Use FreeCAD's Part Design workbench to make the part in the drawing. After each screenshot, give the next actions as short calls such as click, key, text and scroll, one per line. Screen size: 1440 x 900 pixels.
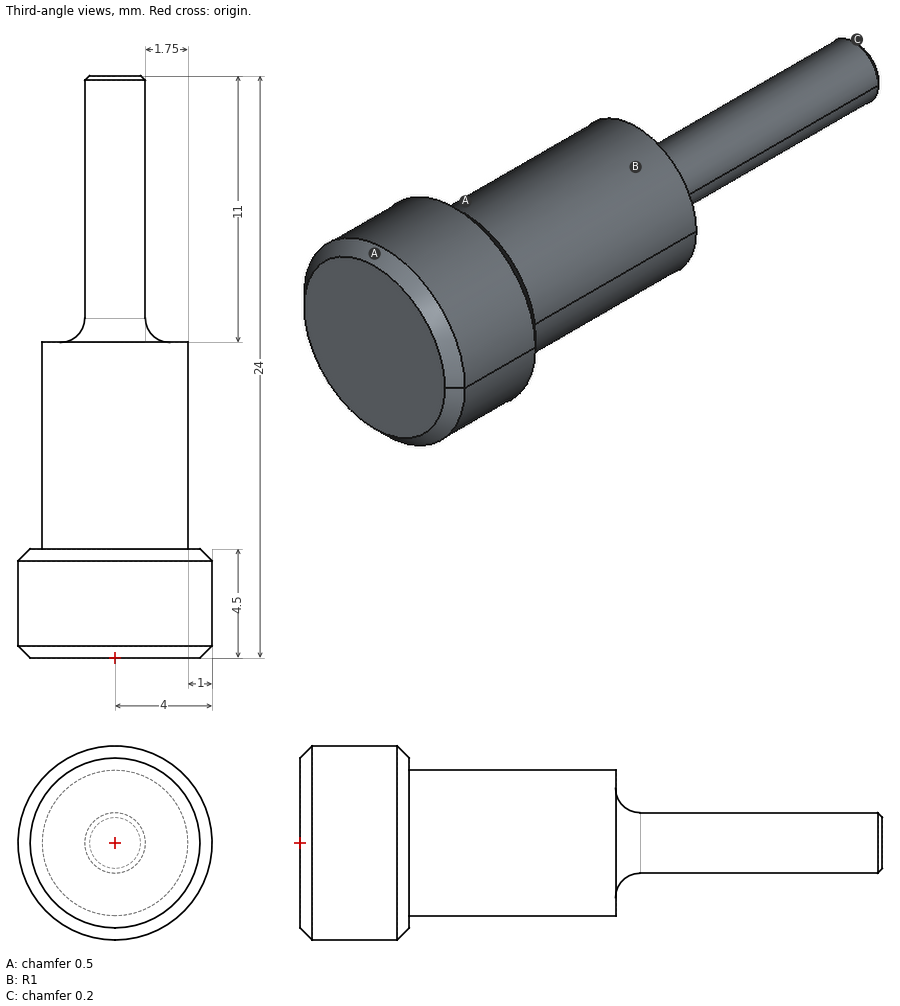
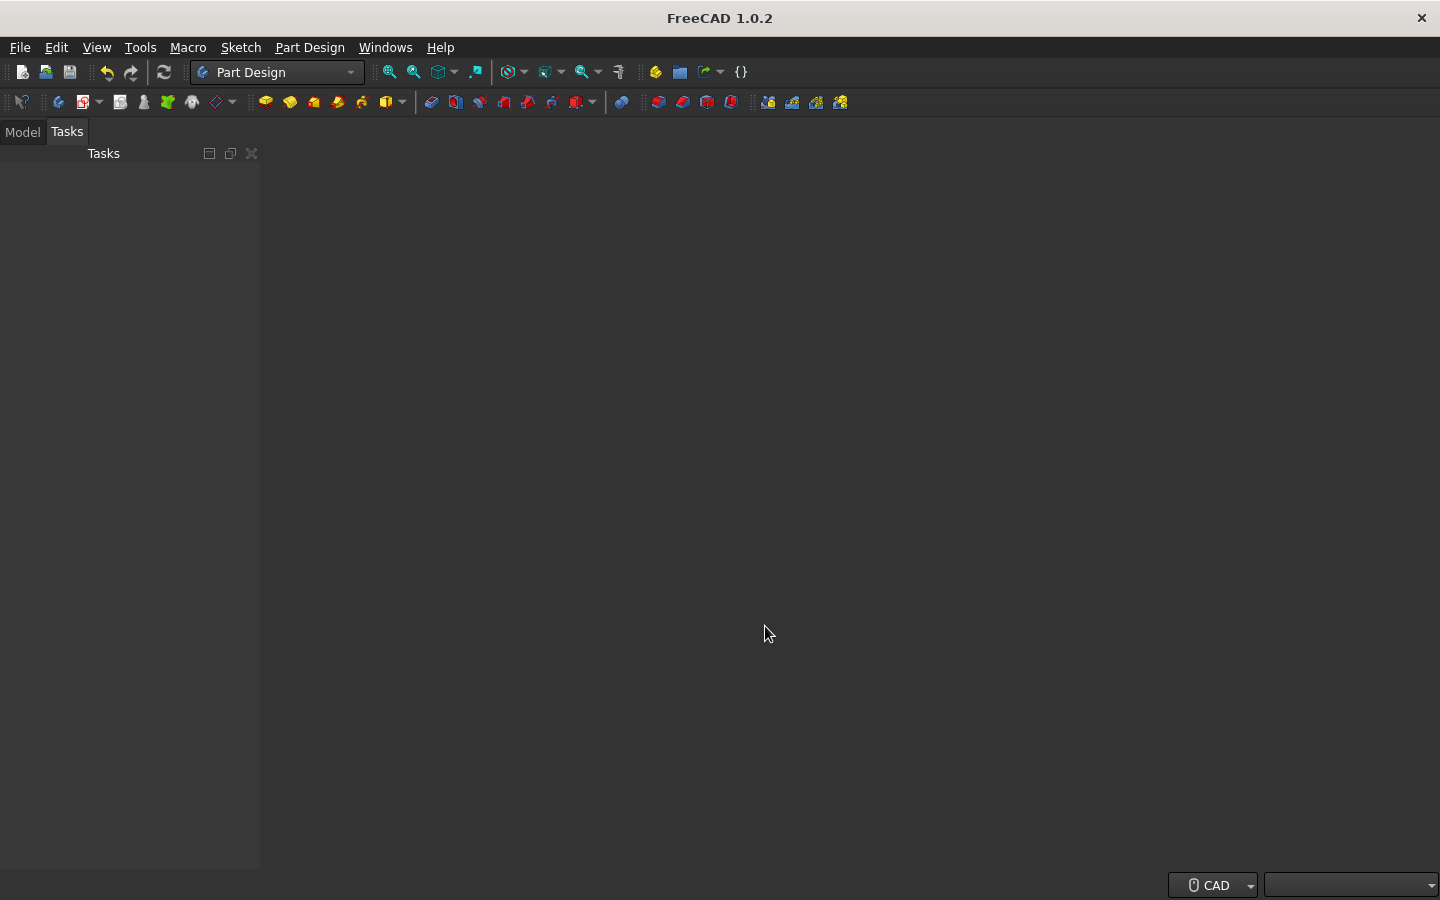
click(22, 72)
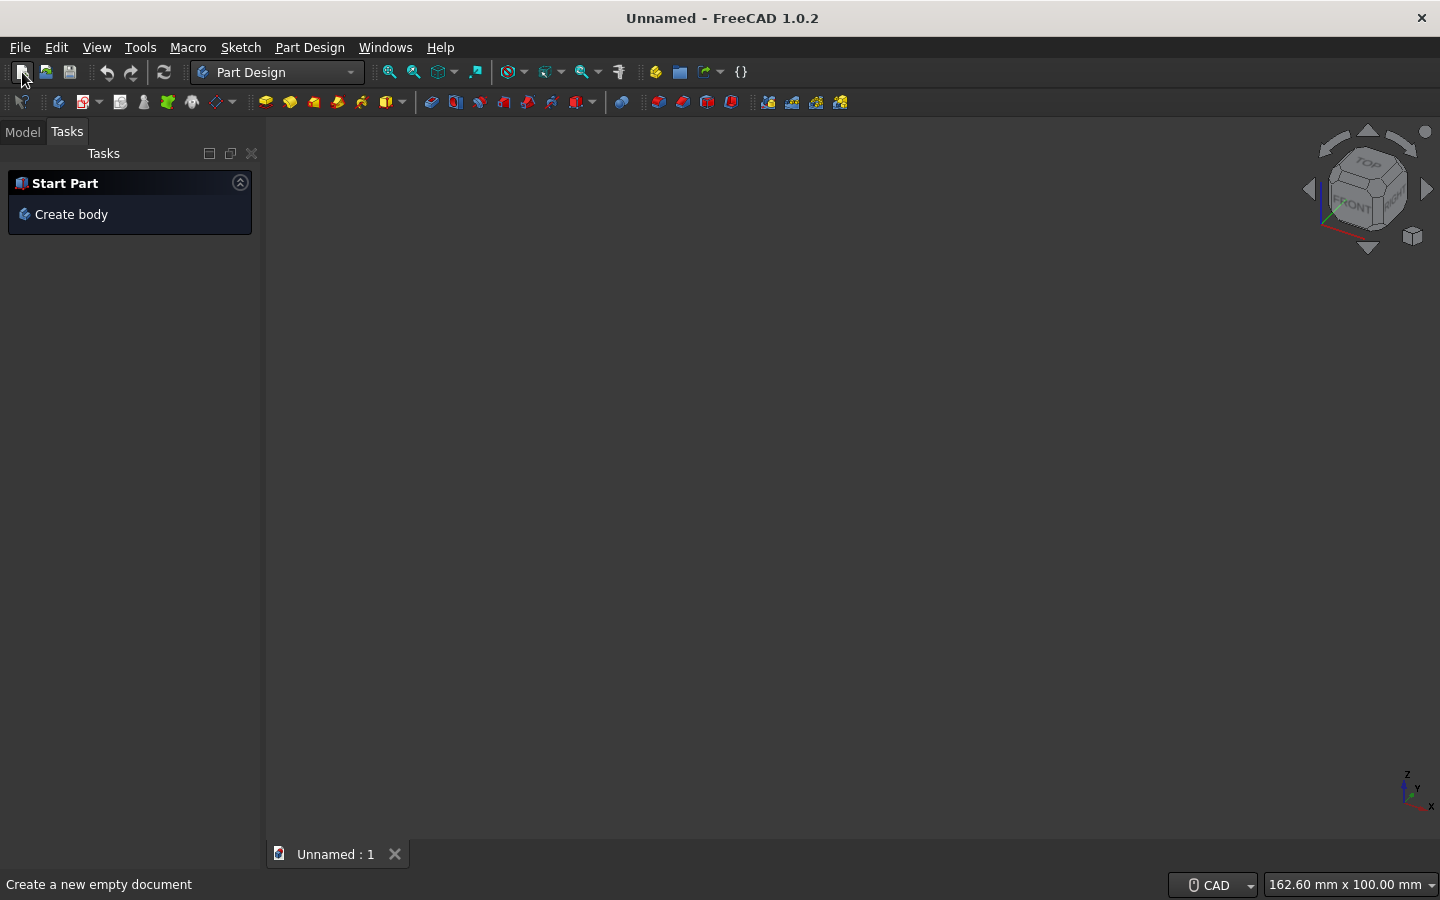
click(84, 102)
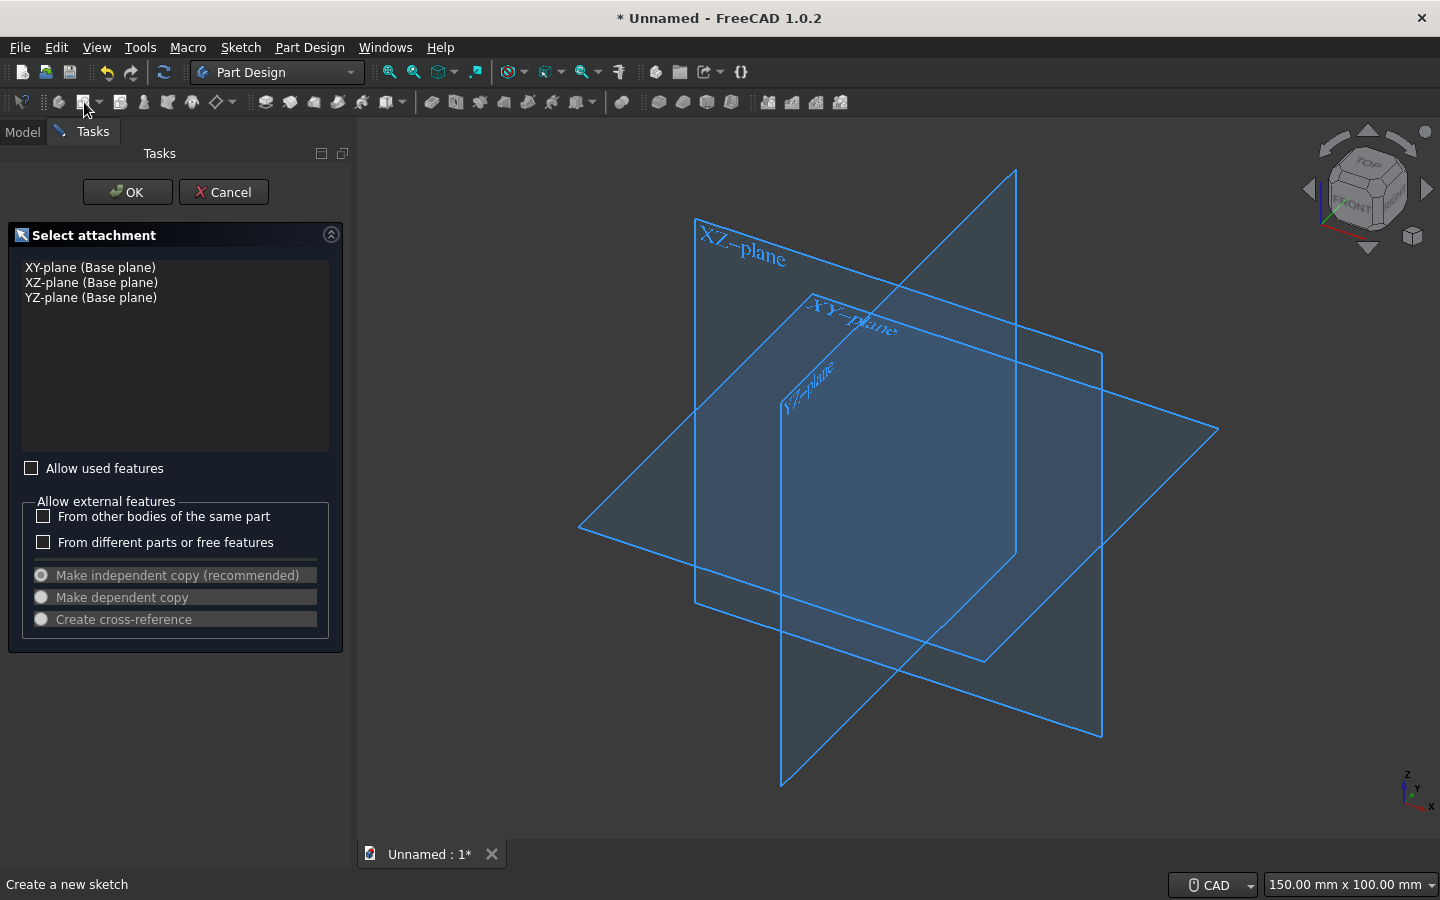
click(82, 268)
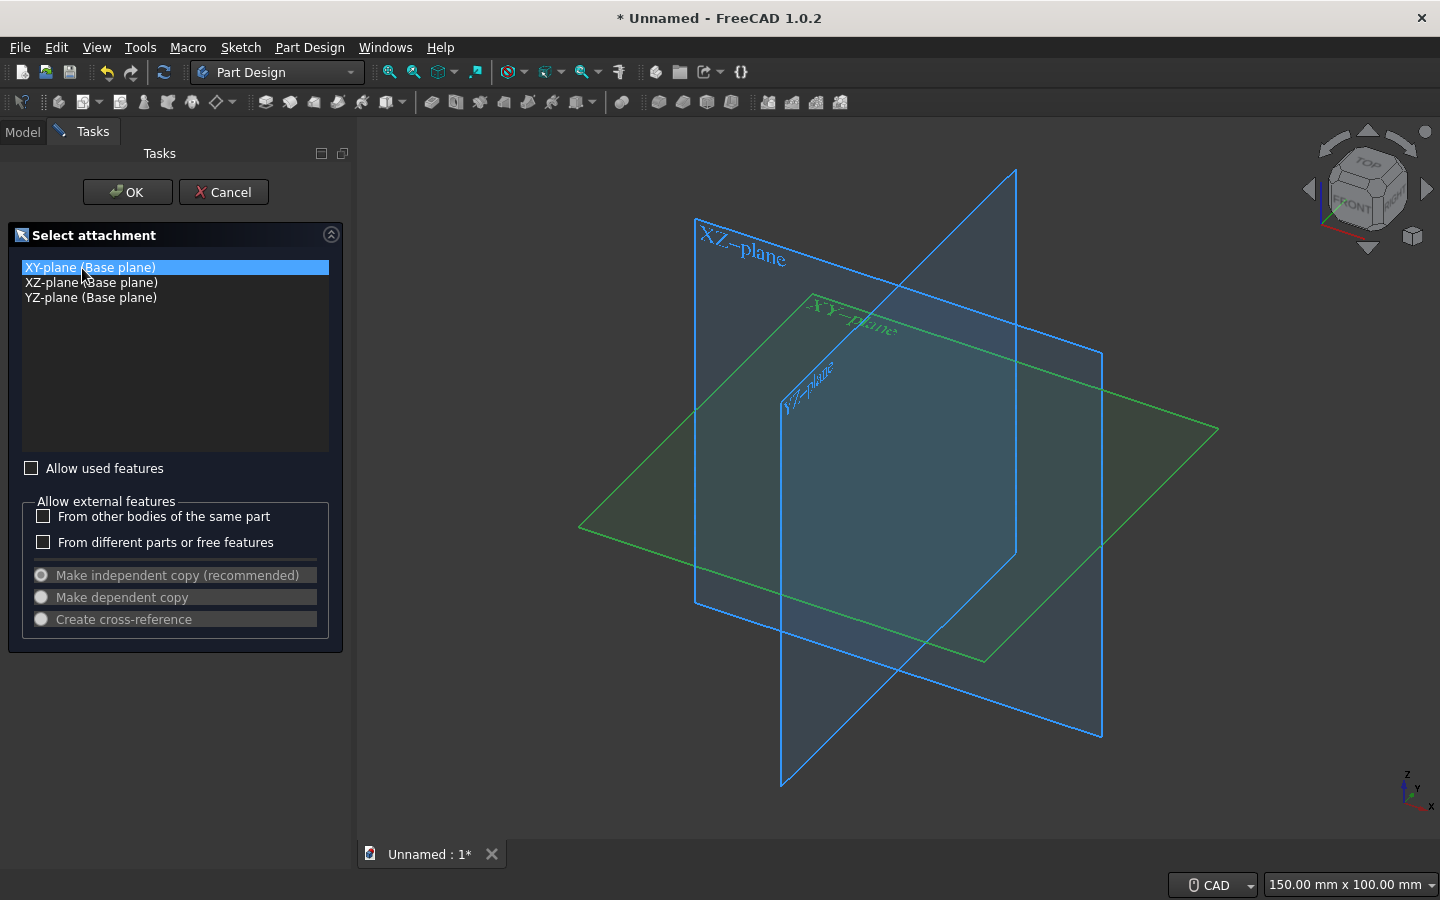
click(128, 192)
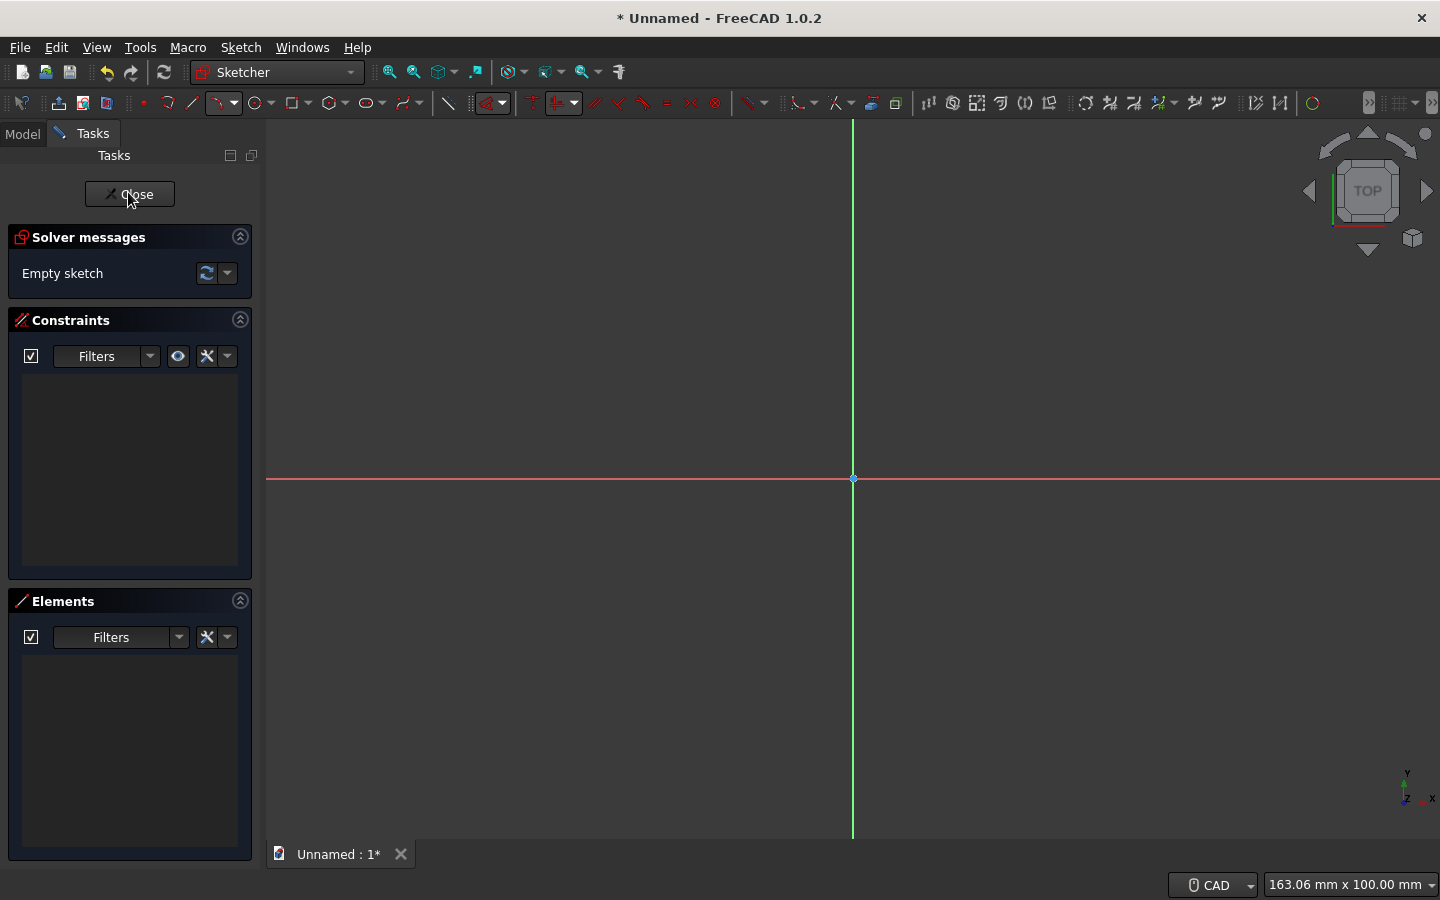
scroll(916, 342, up, 5)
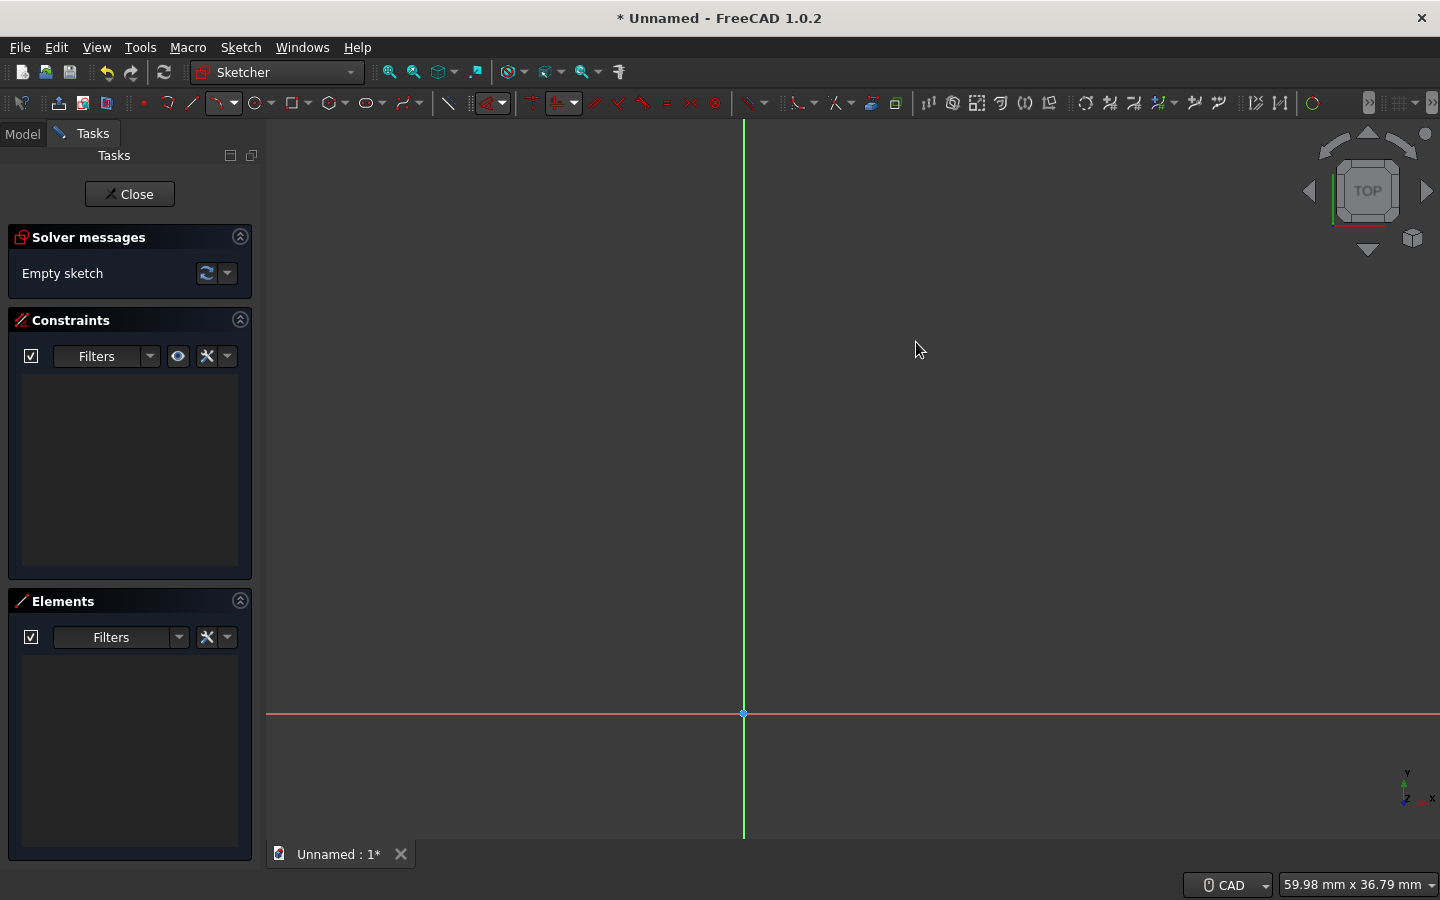
click(168, 104)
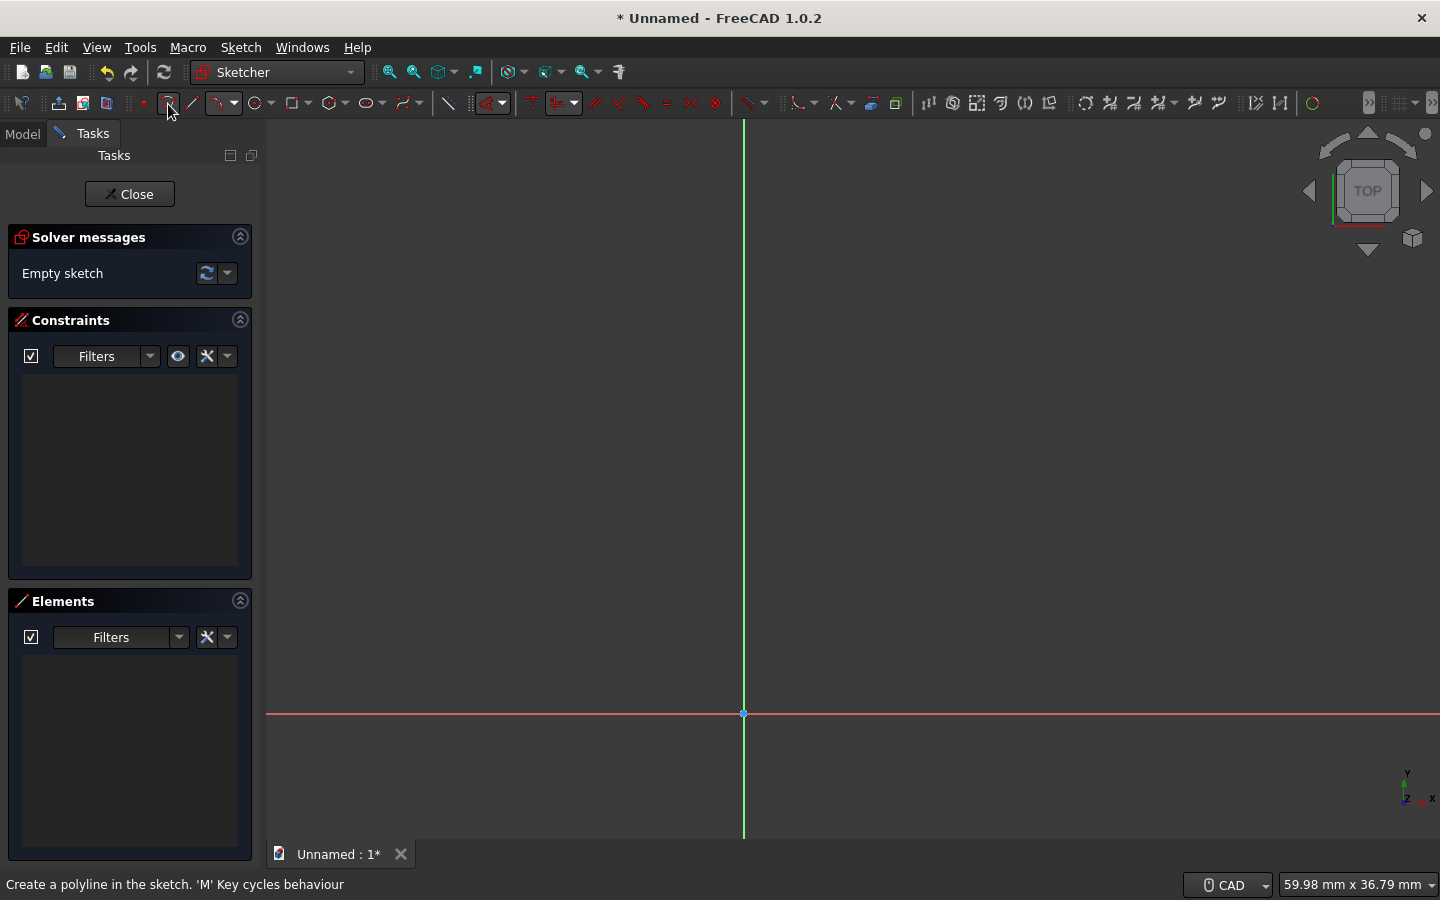
click(744, 714)
click(822, 705)
click(822, 626)
click(803, 626)
click(803, 459)
click(768, 459)
click(768, 244)
click(753, 244)
click(744, 714)
key(Escape)
key(Escape)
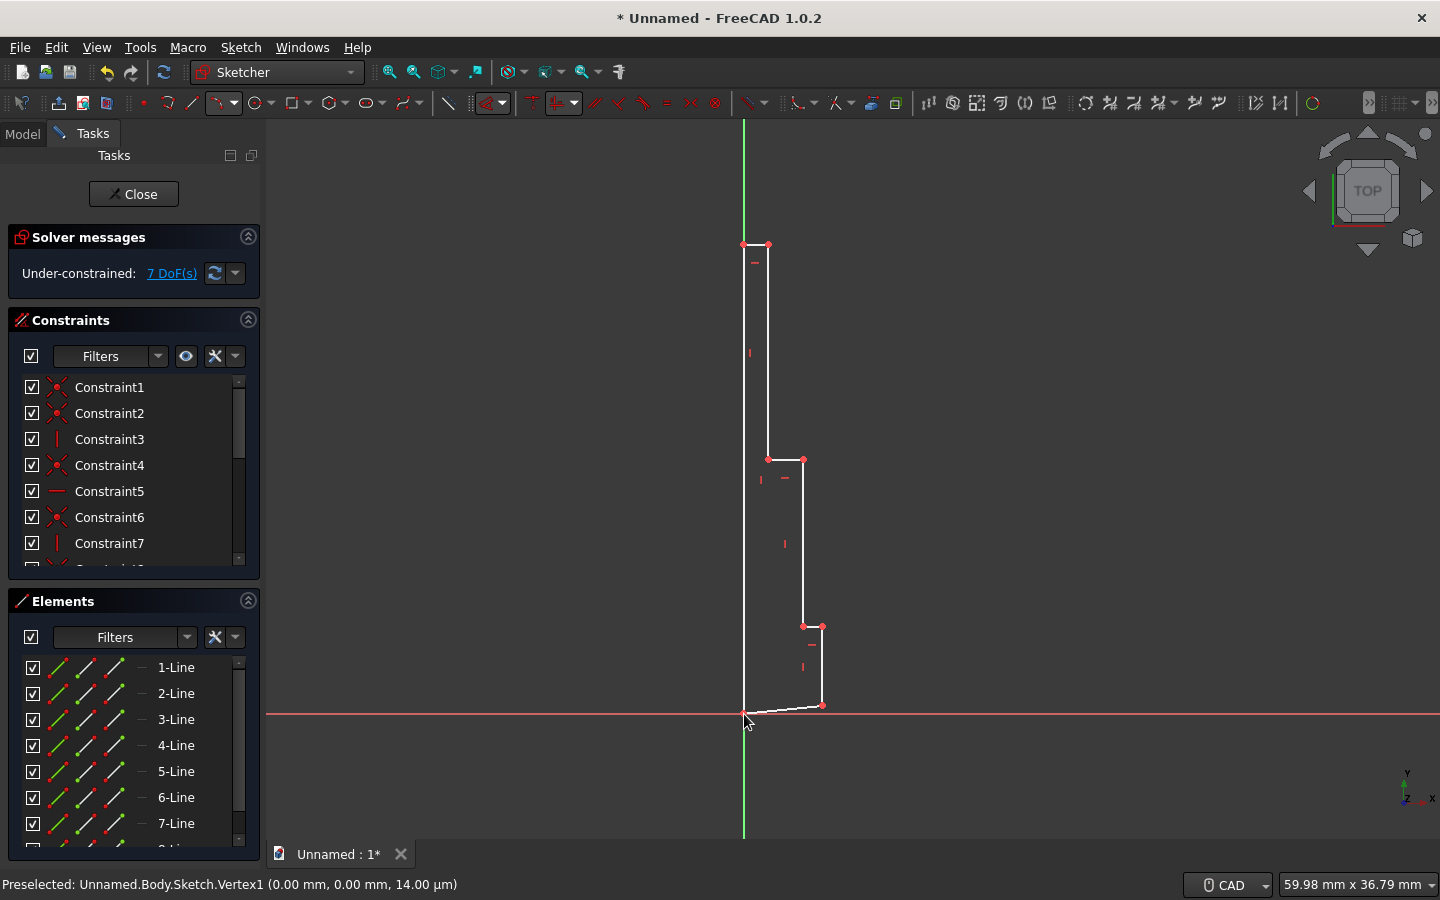
click(767, 712)